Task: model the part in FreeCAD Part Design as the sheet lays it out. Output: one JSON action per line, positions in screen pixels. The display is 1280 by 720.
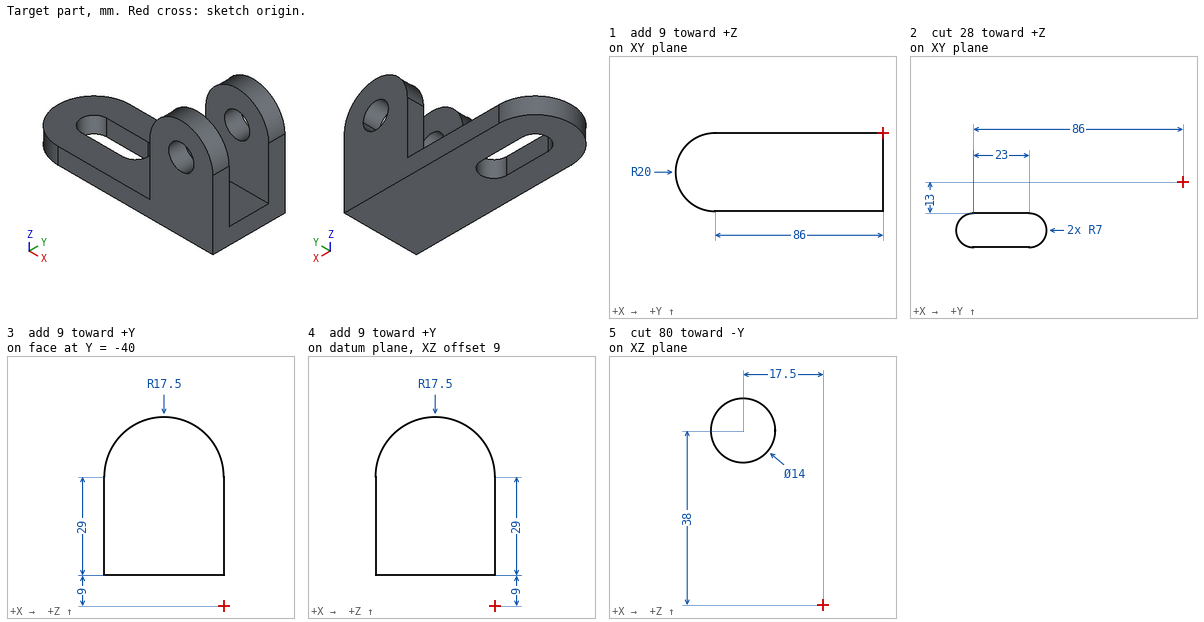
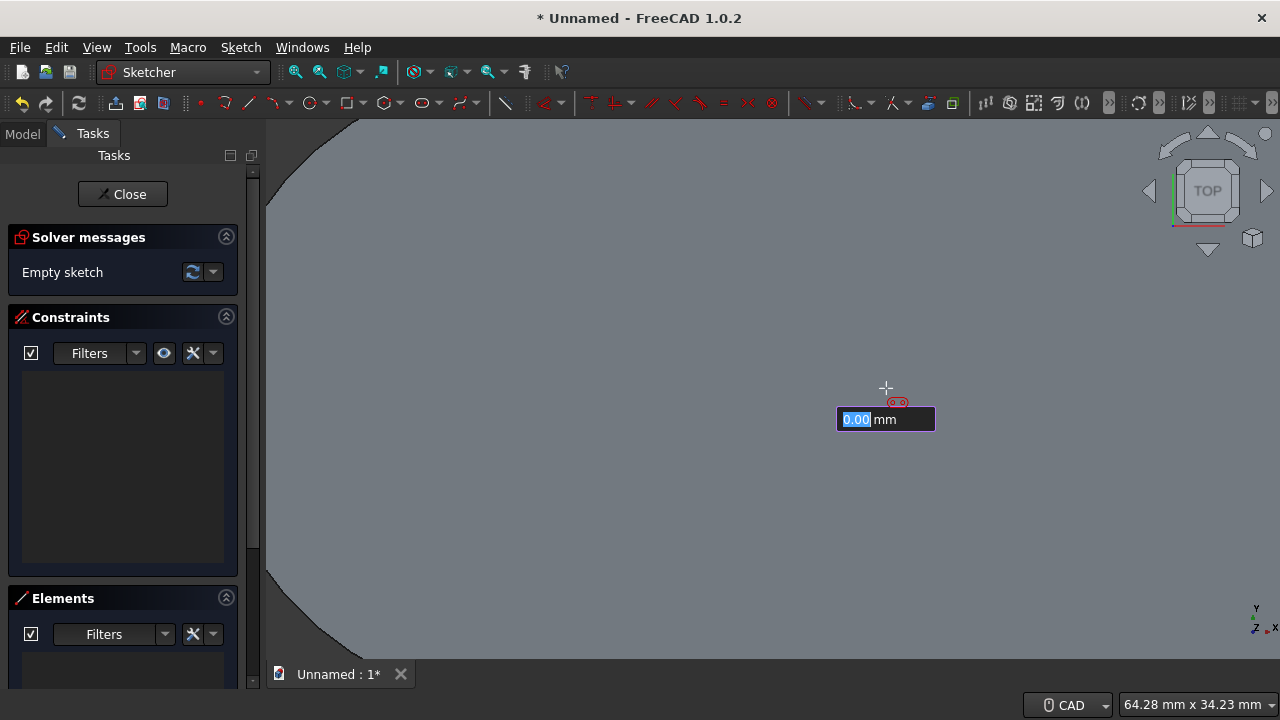
{"action": "left_click", "coordinate": [704, 498]}
{"action": "key", "text": "Escape"}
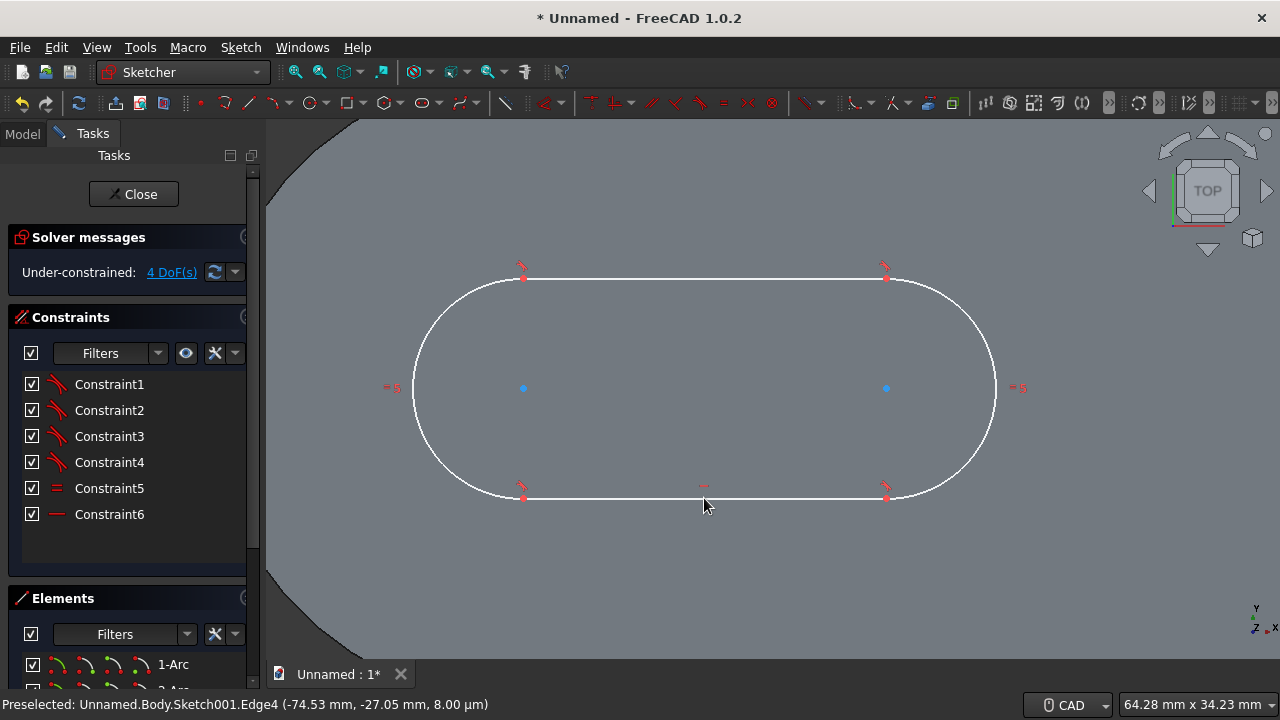
{"action": "left_click", "coordinate": [544, 104]}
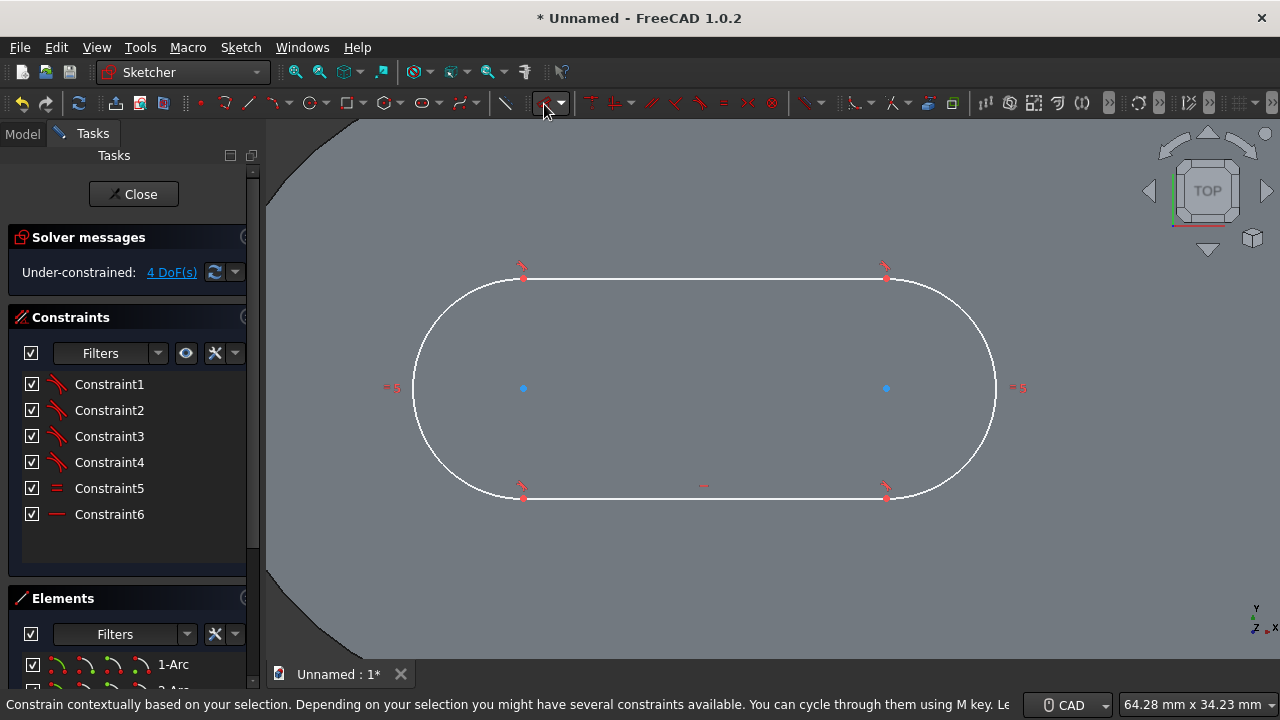
{"action": "left_click", "coordinate": [434, 324]}
{"action": "left_click", "coordinate": [408, 305]}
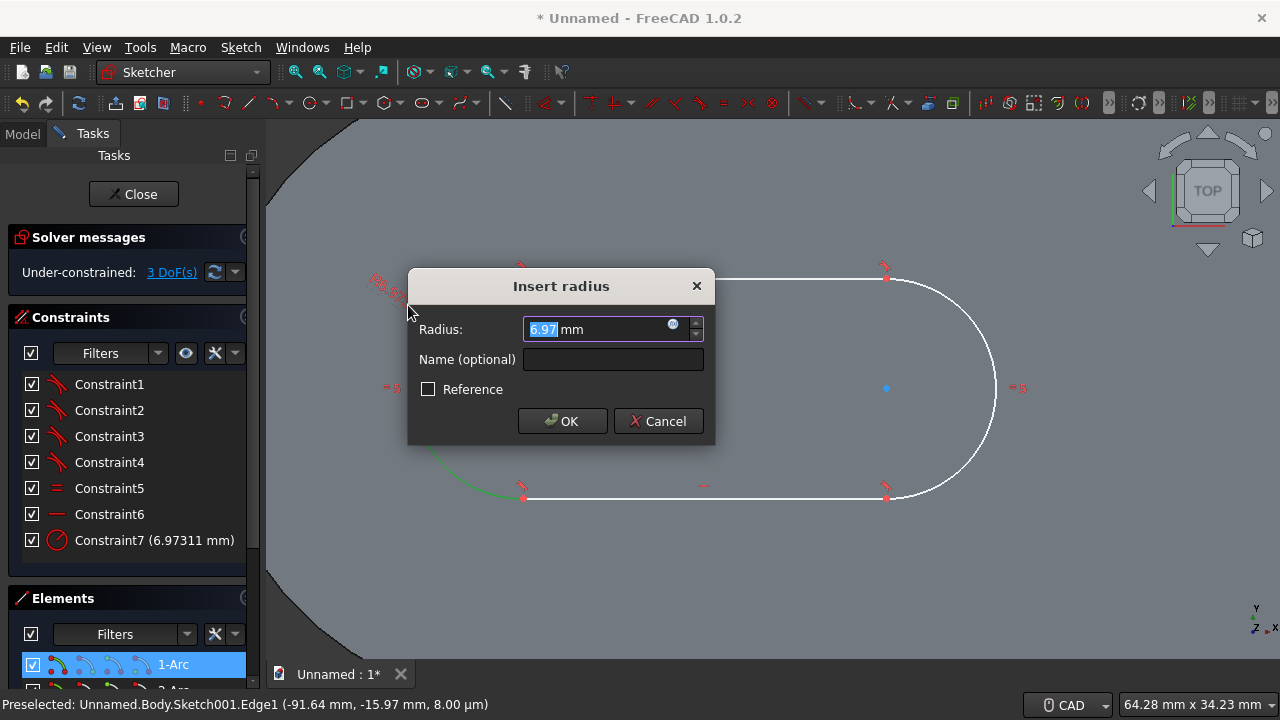
{"action": "type", "text": "7"}
{"action": "key", "text": "Return"}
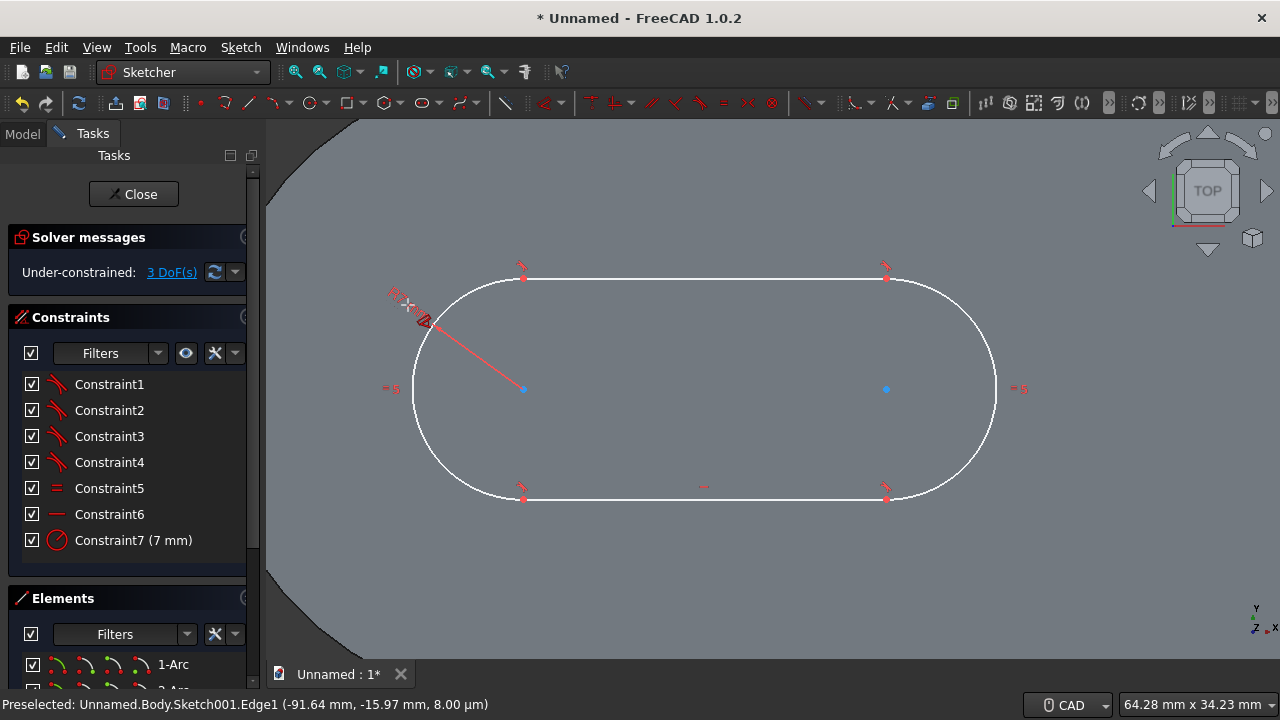
{"action": "left_click", "coordinate": [632, 279]}
{"action": "left_click", "coordinate": [704, 245]}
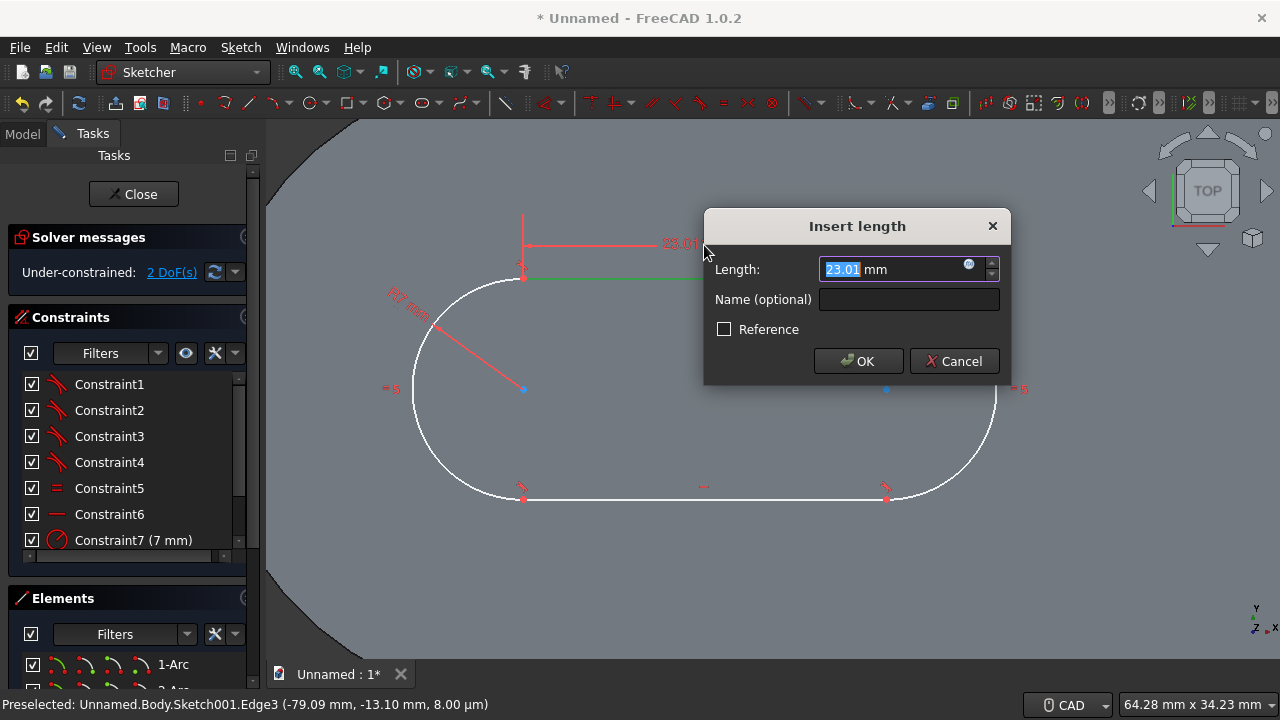
{"action": "type", "text": "23"}
{"action": "key", "text": "Return"}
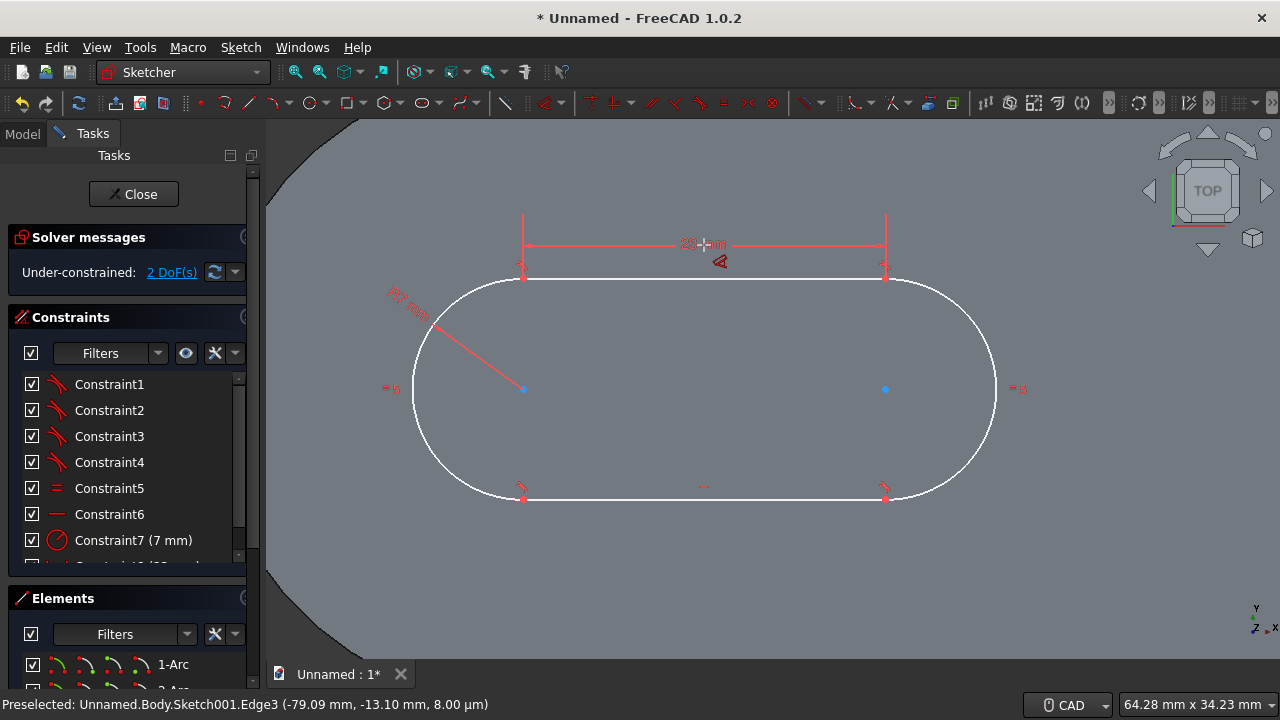
{"action": "left_click", "coordinate": [523, 279]}
{"action": "left_click", "coordinate": [819, 313]}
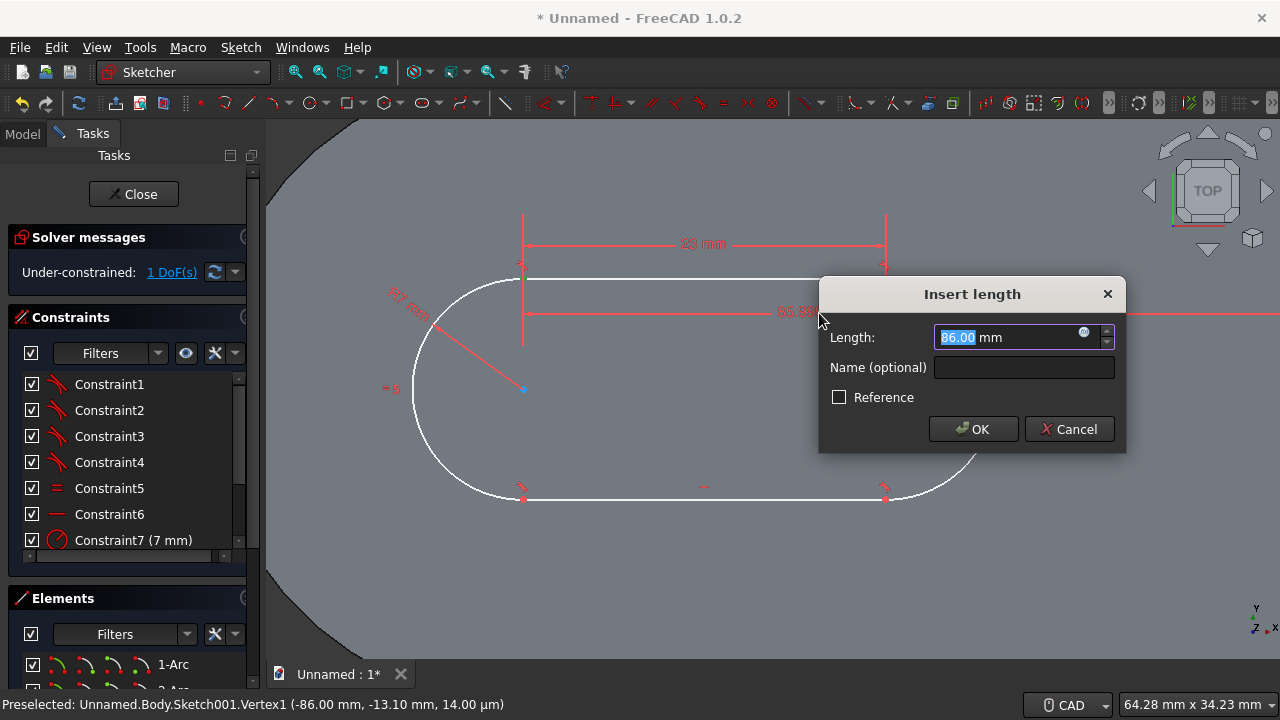
{"action": "type", "text": "86"}
{"action": "key", "text": "Return"}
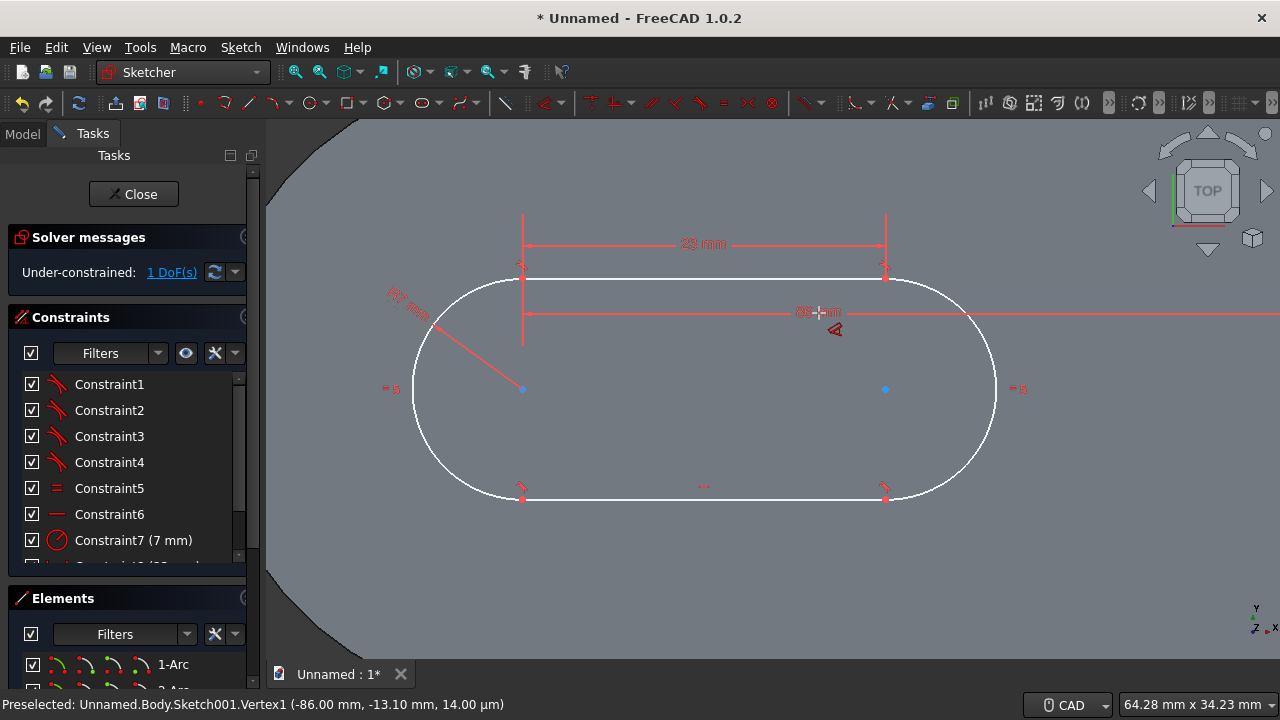
{"action": "left_click", "coordinate": [523, 279]}
{"action": "left_click", "coordinate": [489, 213]}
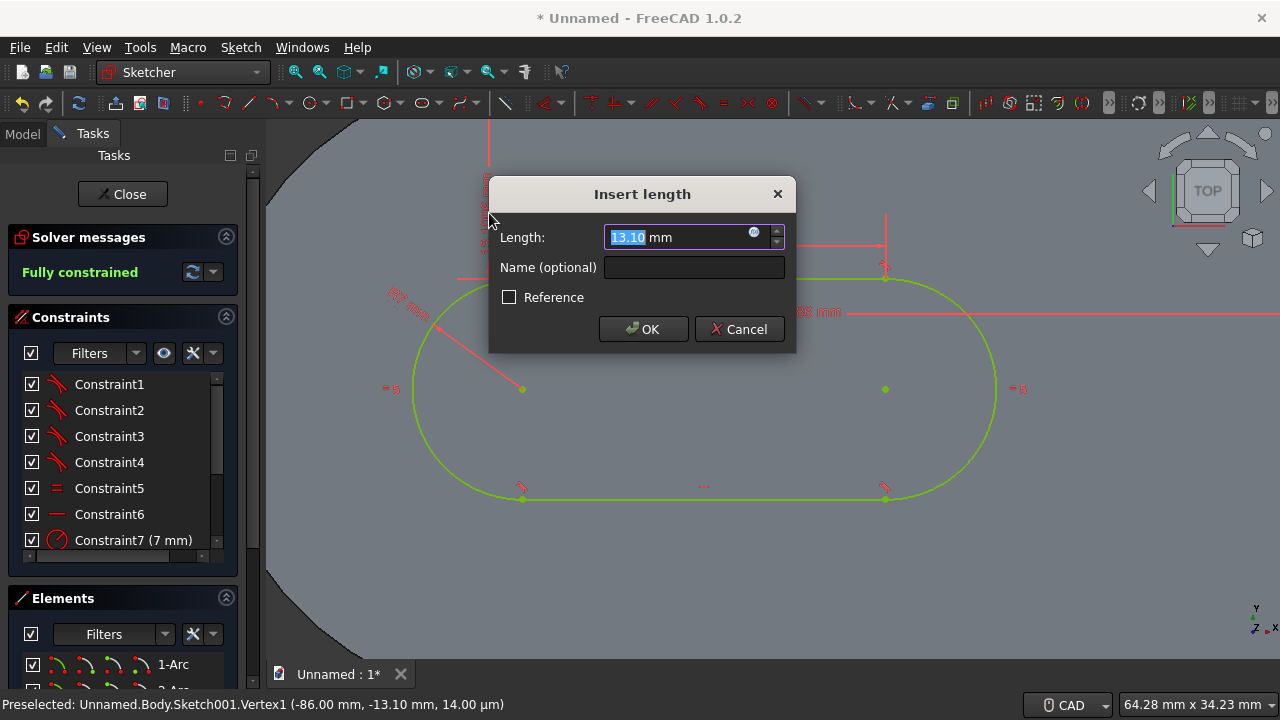
{"action": "type", "text": "13"}
{"action": "key", "text": "Return"}
{"action": "key", "text": "Escape"}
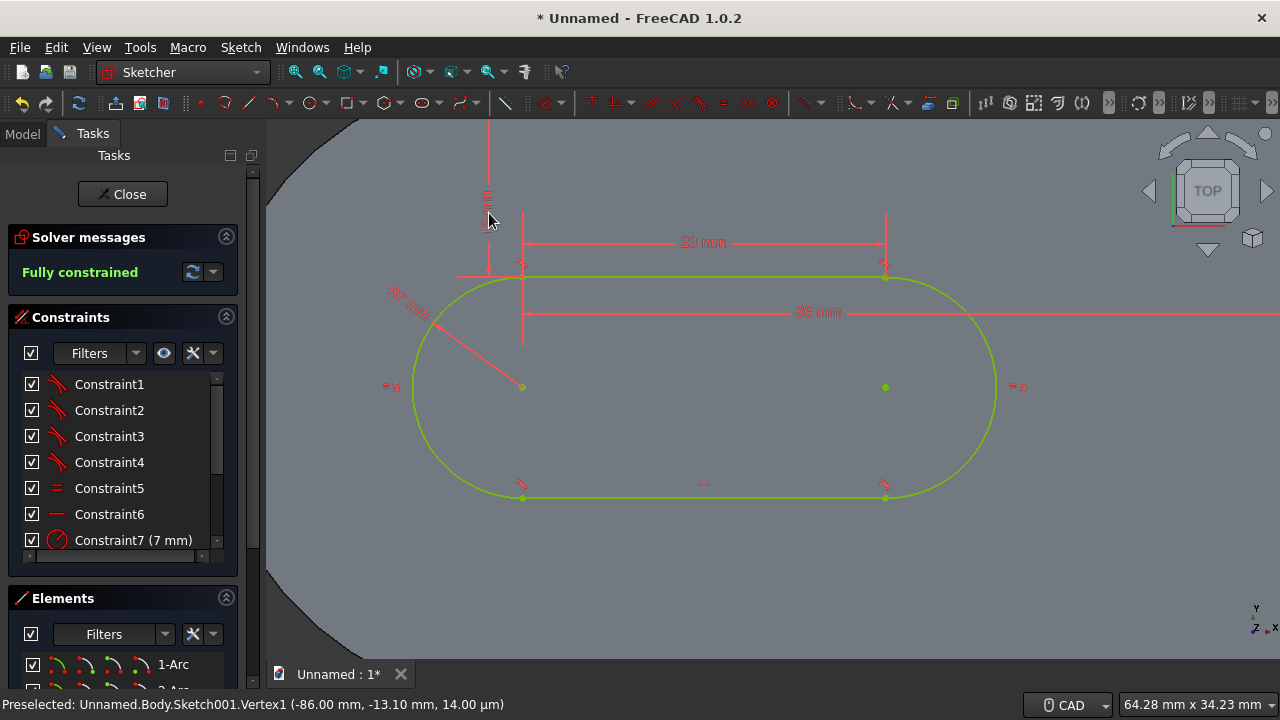
{"action": "left_click", "coordinate": [123, 194]}